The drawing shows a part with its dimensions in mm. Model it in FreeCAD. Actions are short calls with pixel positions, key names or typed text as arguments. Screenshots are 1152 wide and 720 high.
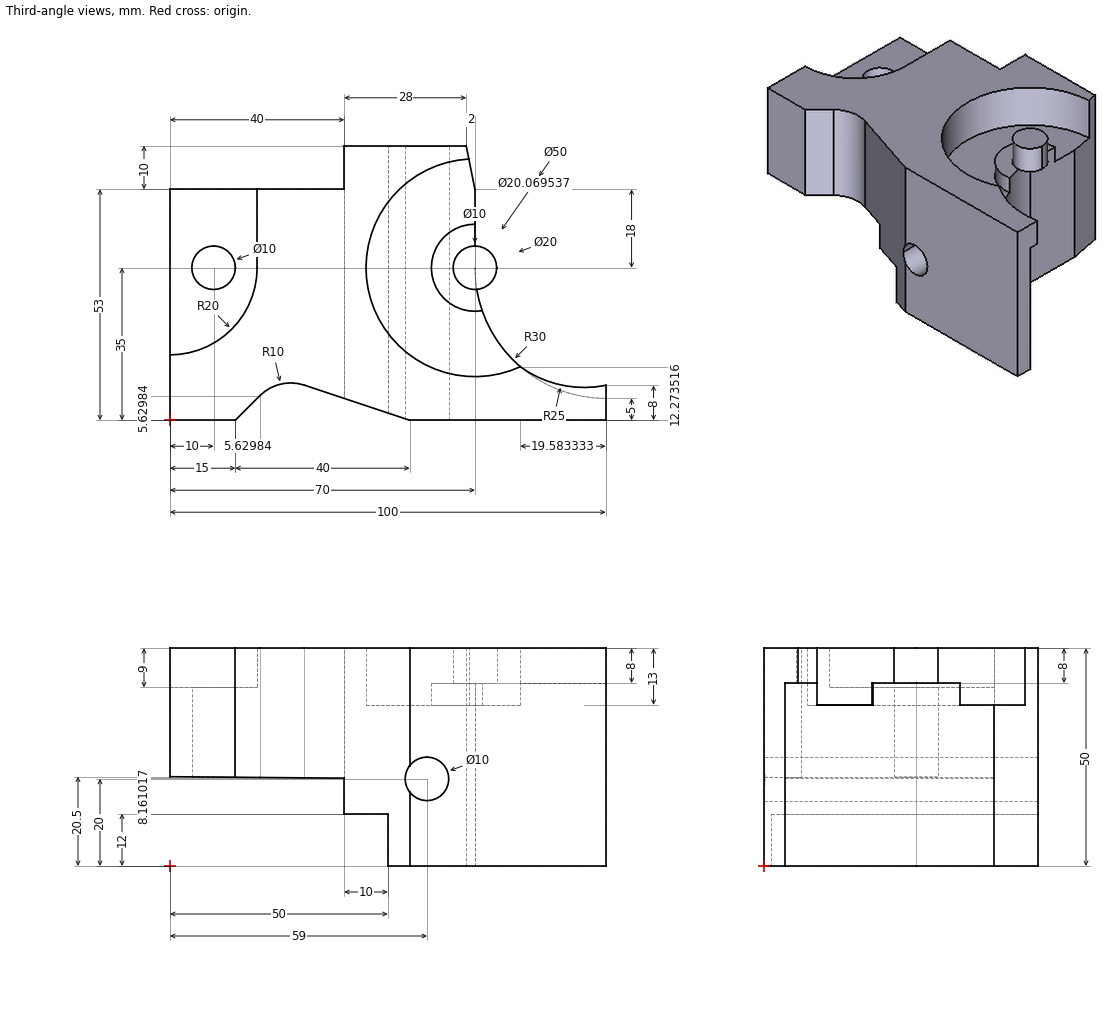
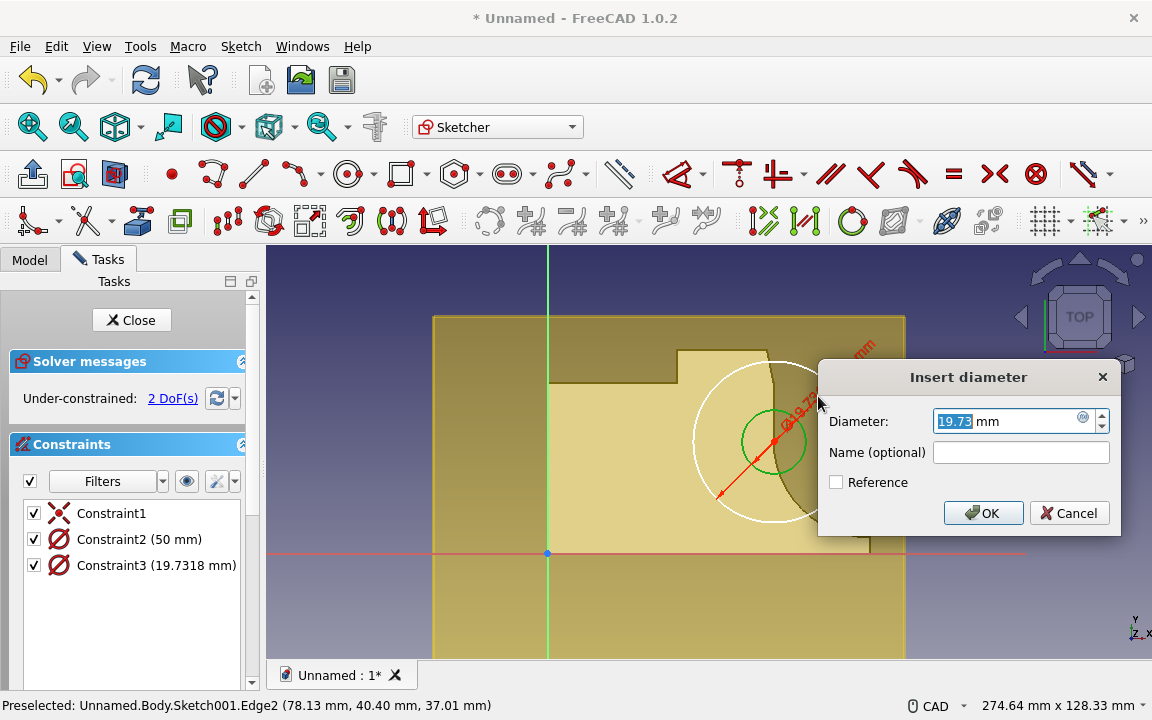
text(20)
key(Return)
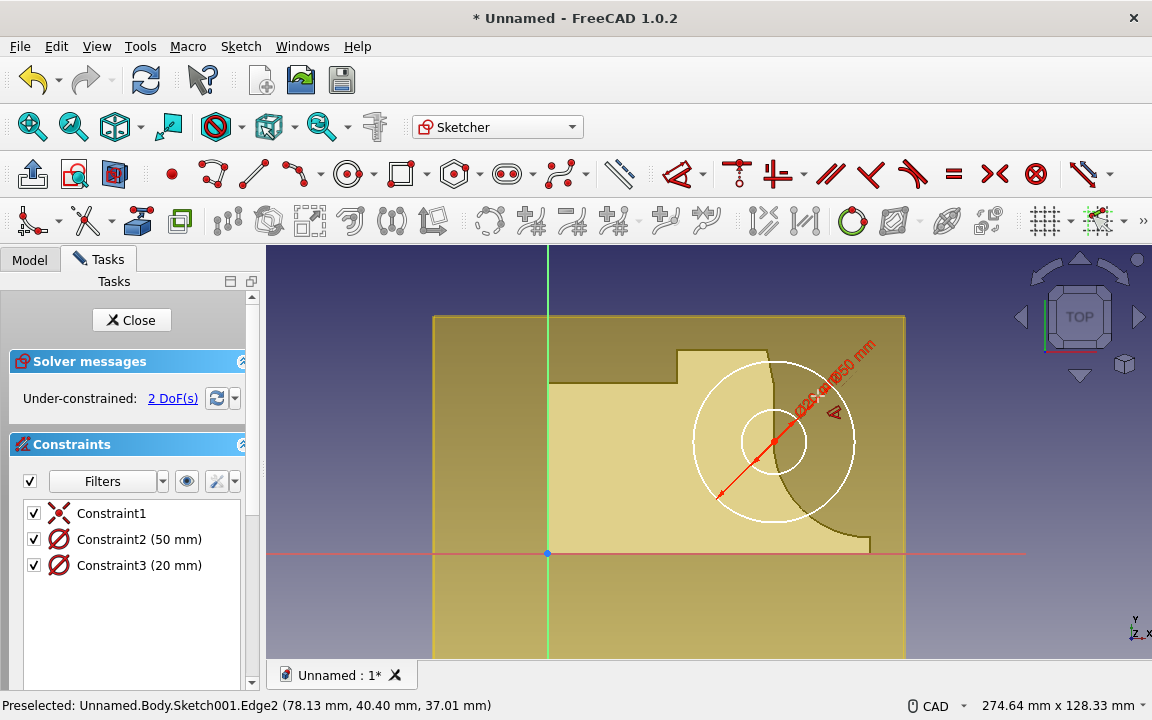
click(774, 442)
click(661, 588)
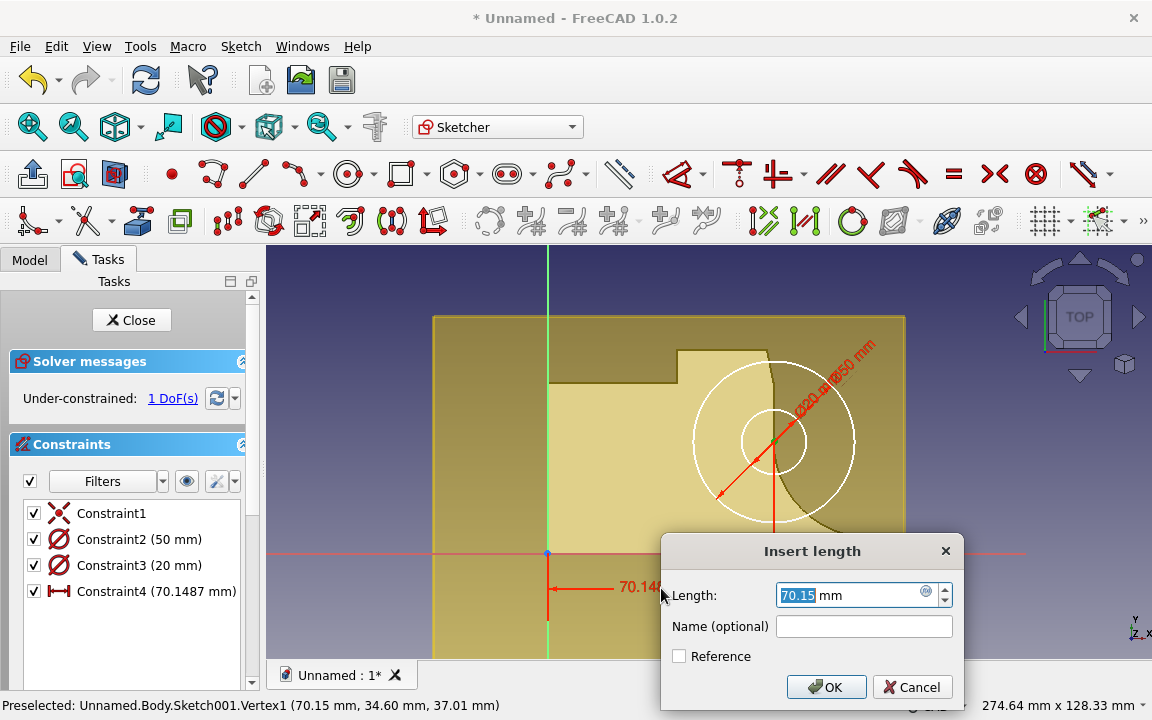
text(70)
key(Return)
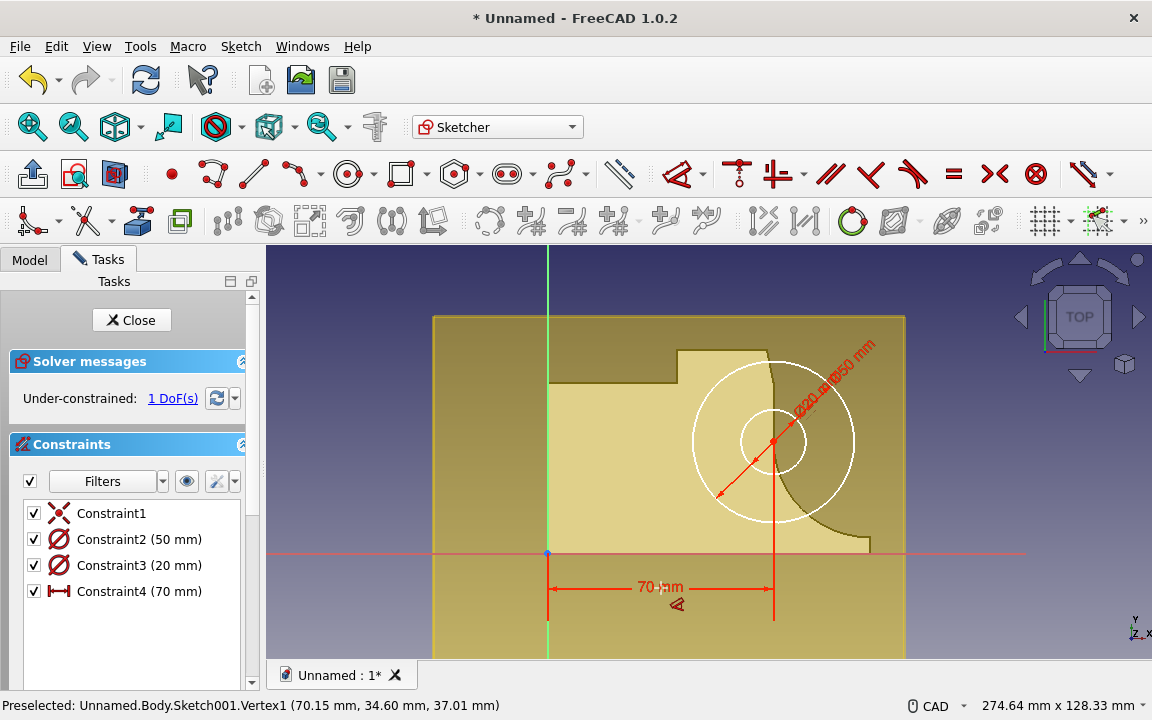
click(774, 442)
click(514, 498)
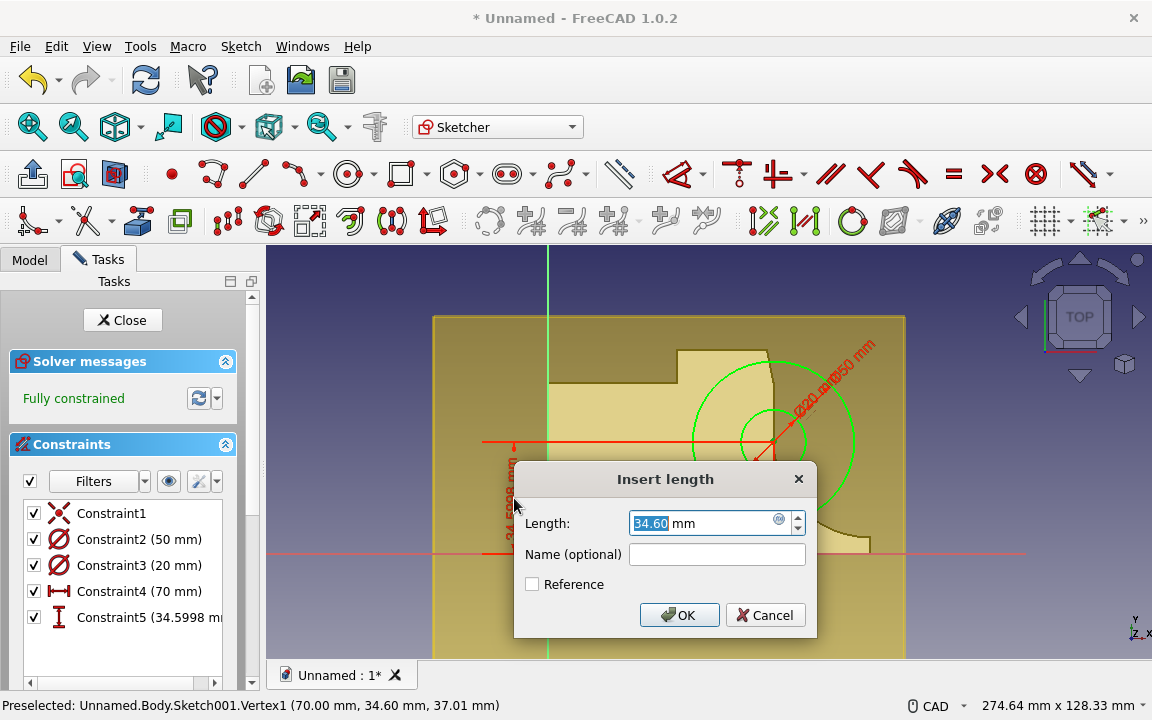
text(35)
key(Return)
key(Escape)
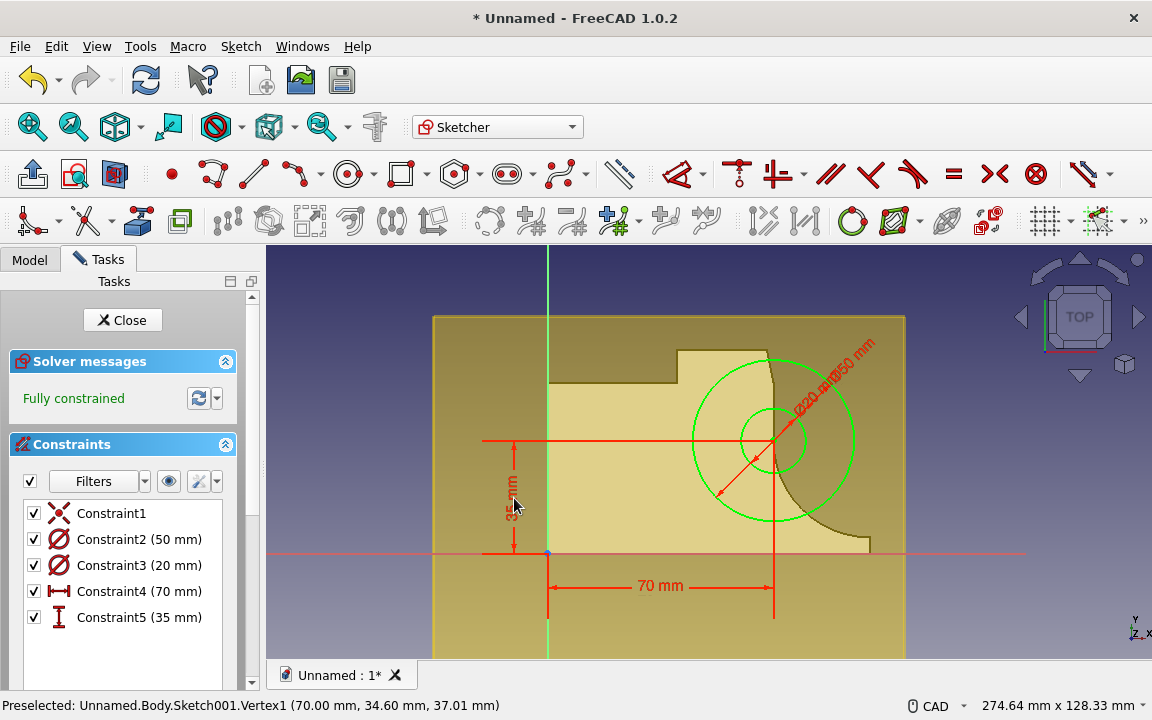
click(123, 320)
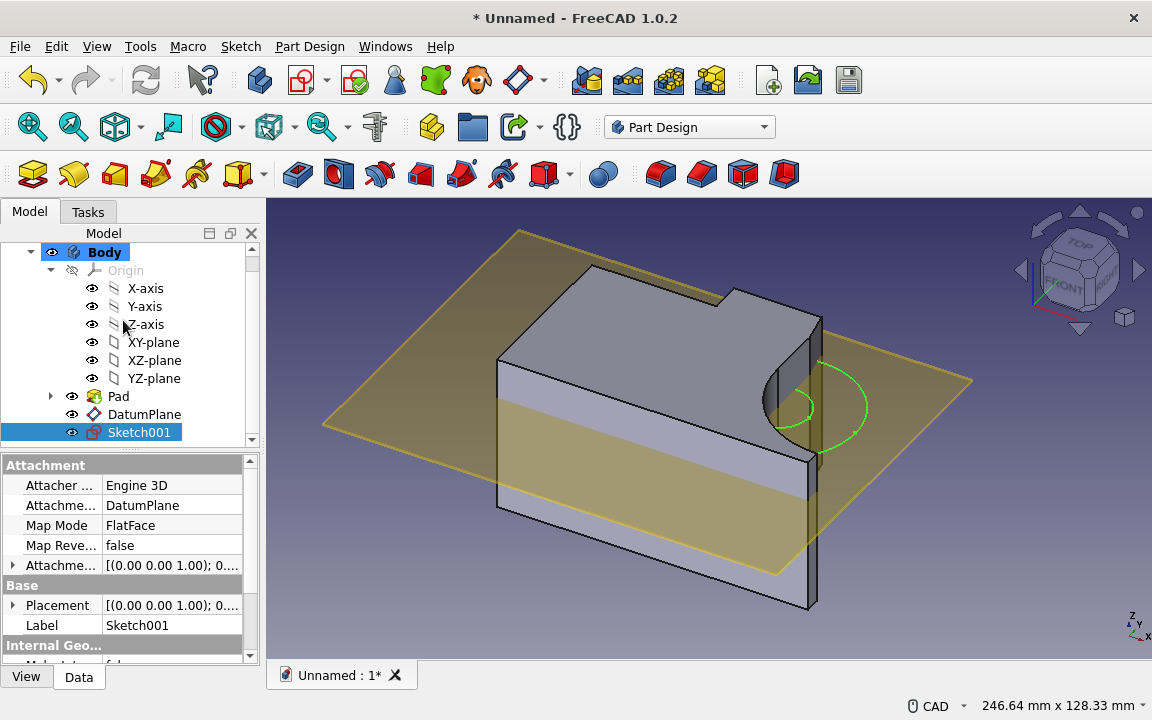
click(298, 174)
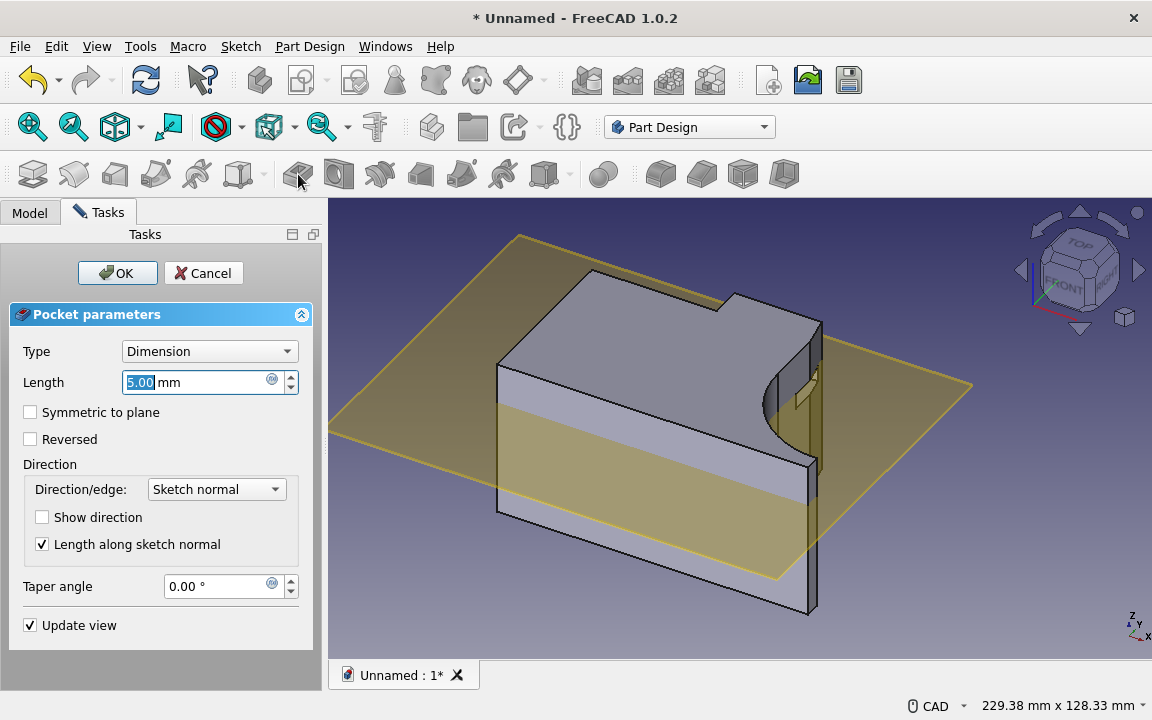
text(13)
key(Tab)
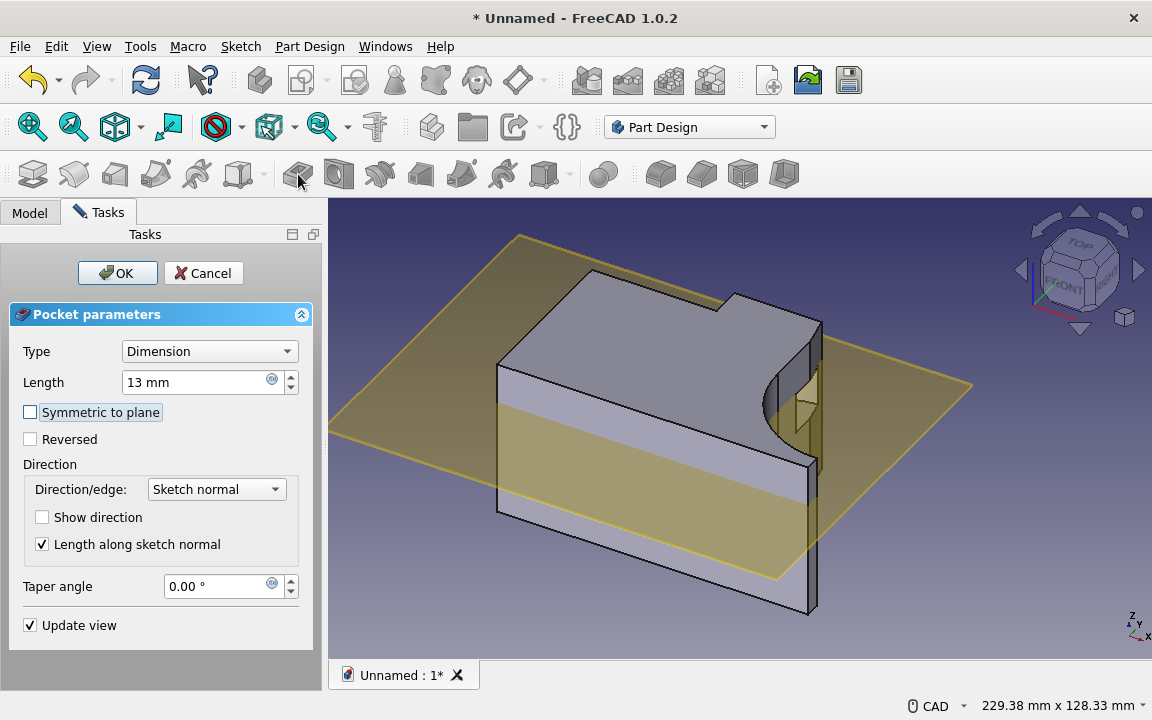
click(31, 439)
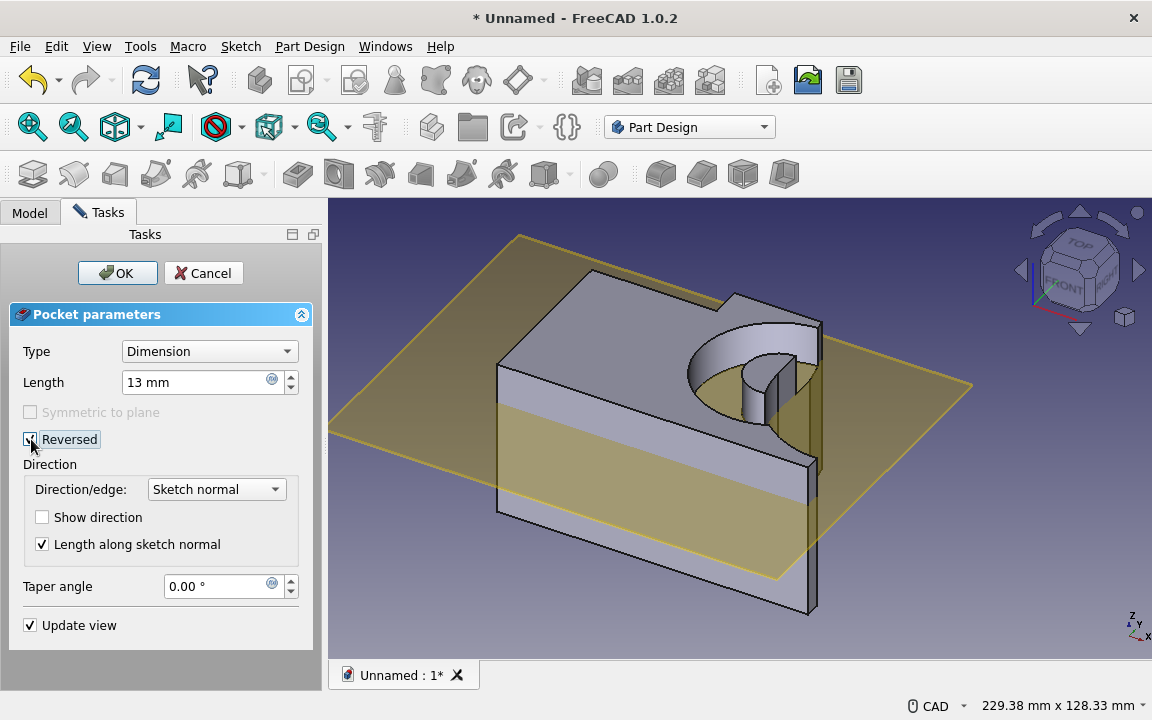
click(118, 273)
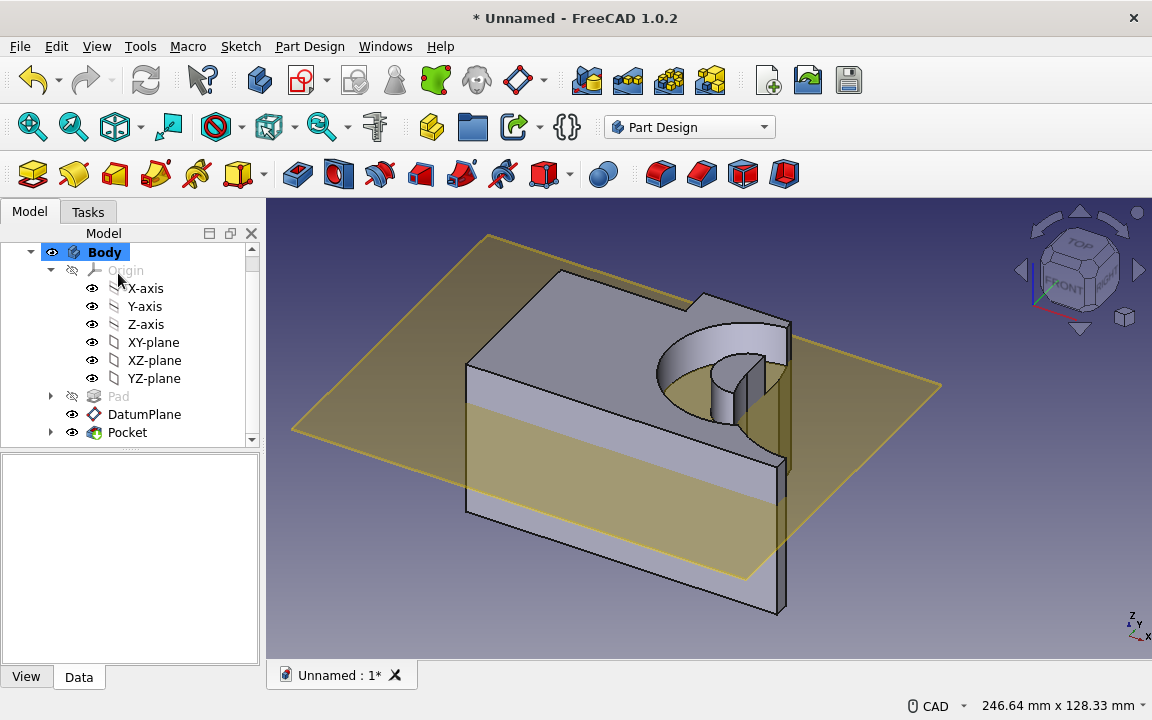
click(117, 414)
key(space)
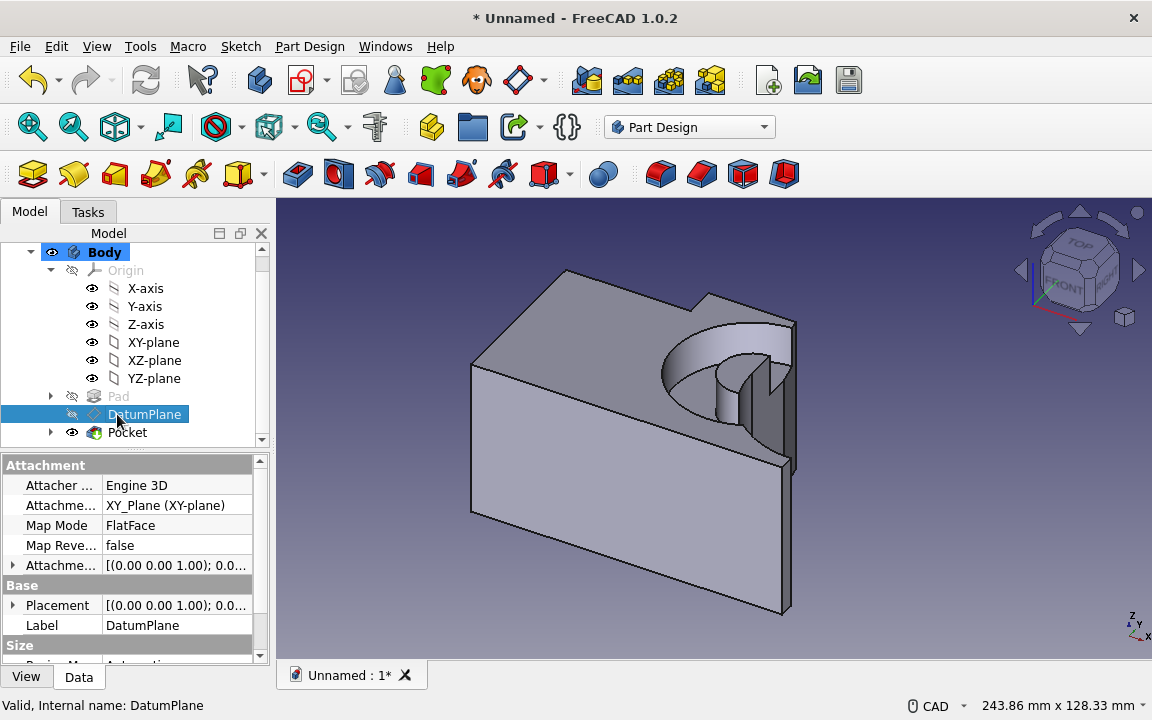
click(594, 329)